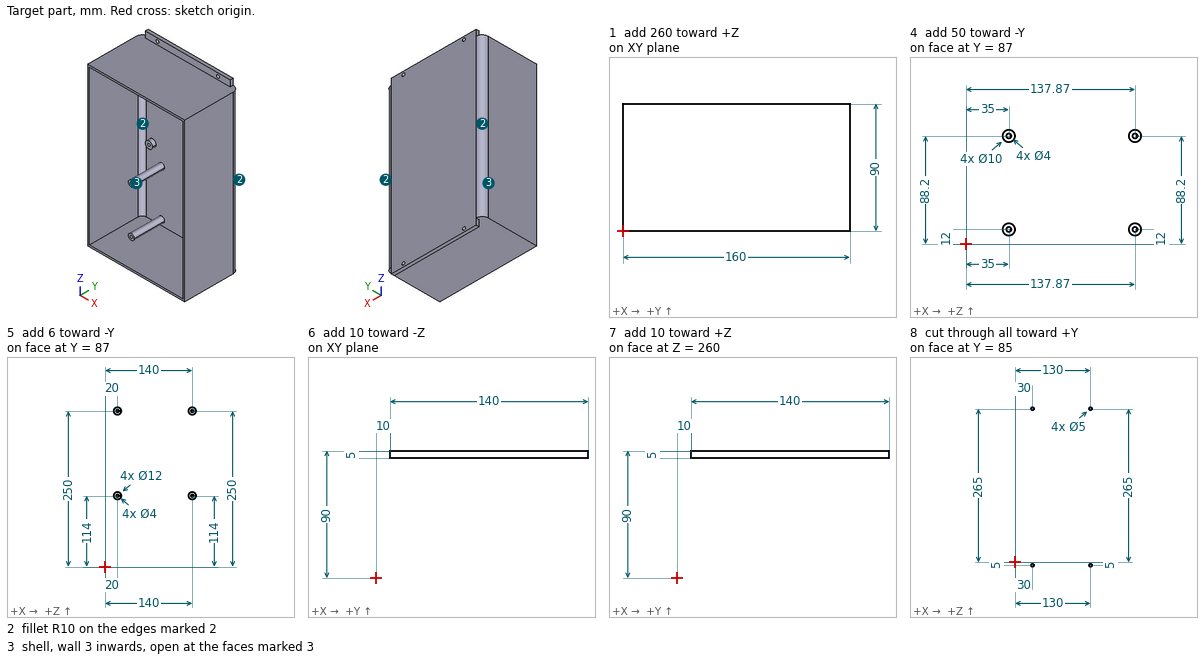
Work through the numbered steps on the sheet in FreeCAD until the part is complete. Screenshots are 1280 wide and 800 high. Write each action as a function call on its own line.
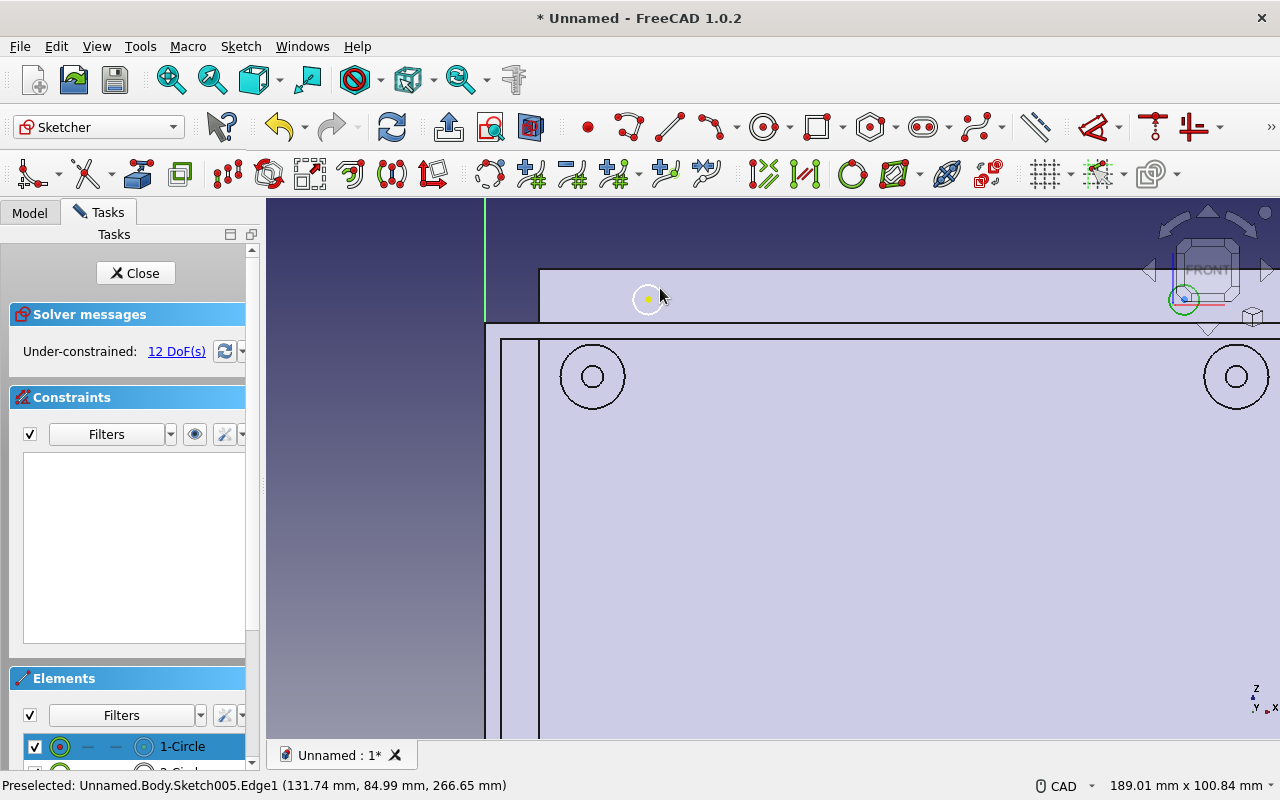
click(658, 289)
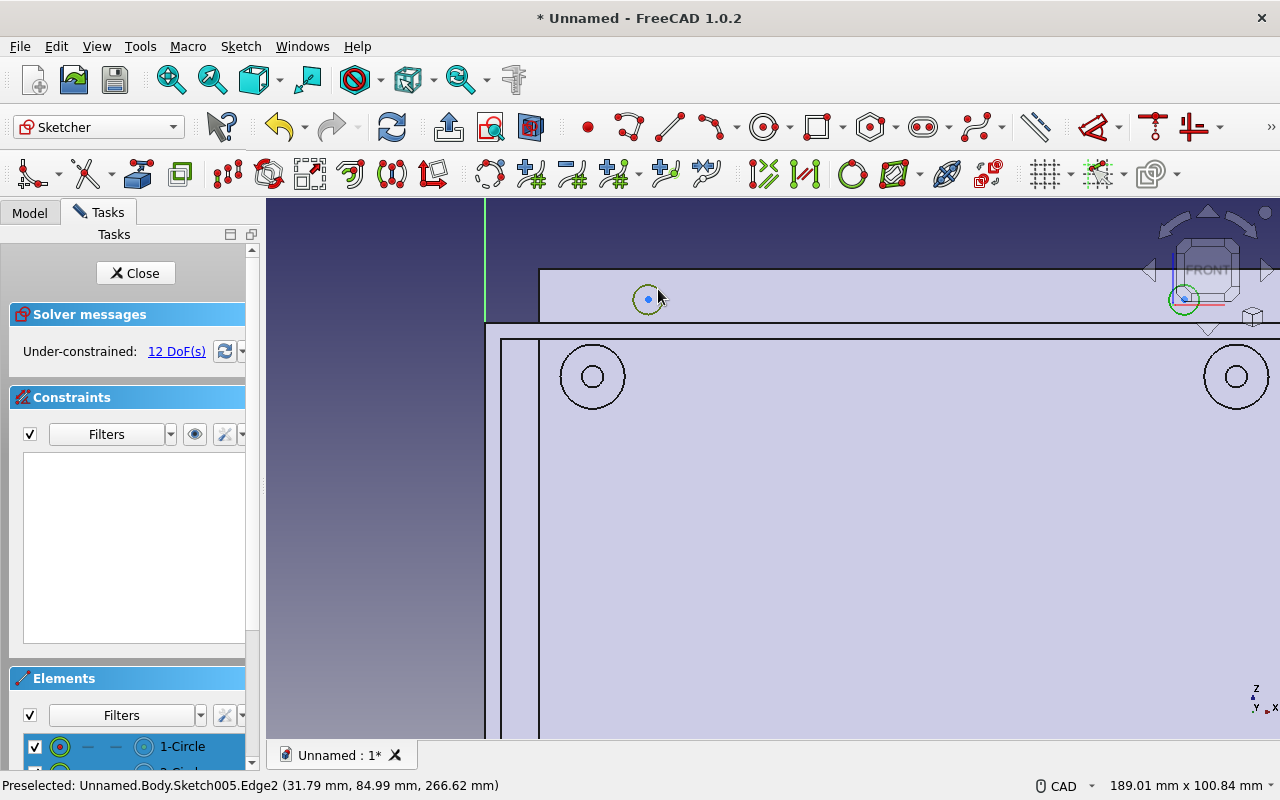
scroll(660, 288, down, 7)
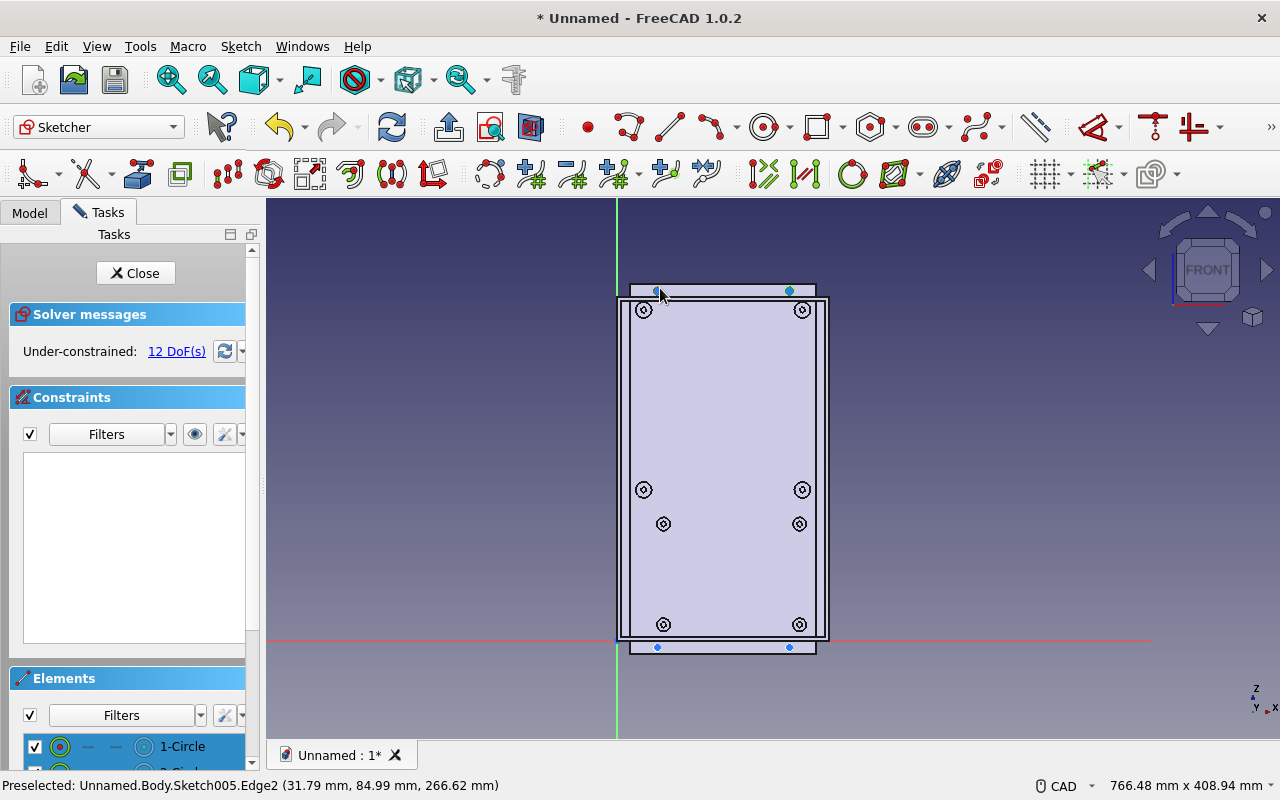
scroll(792, 645, up, 8)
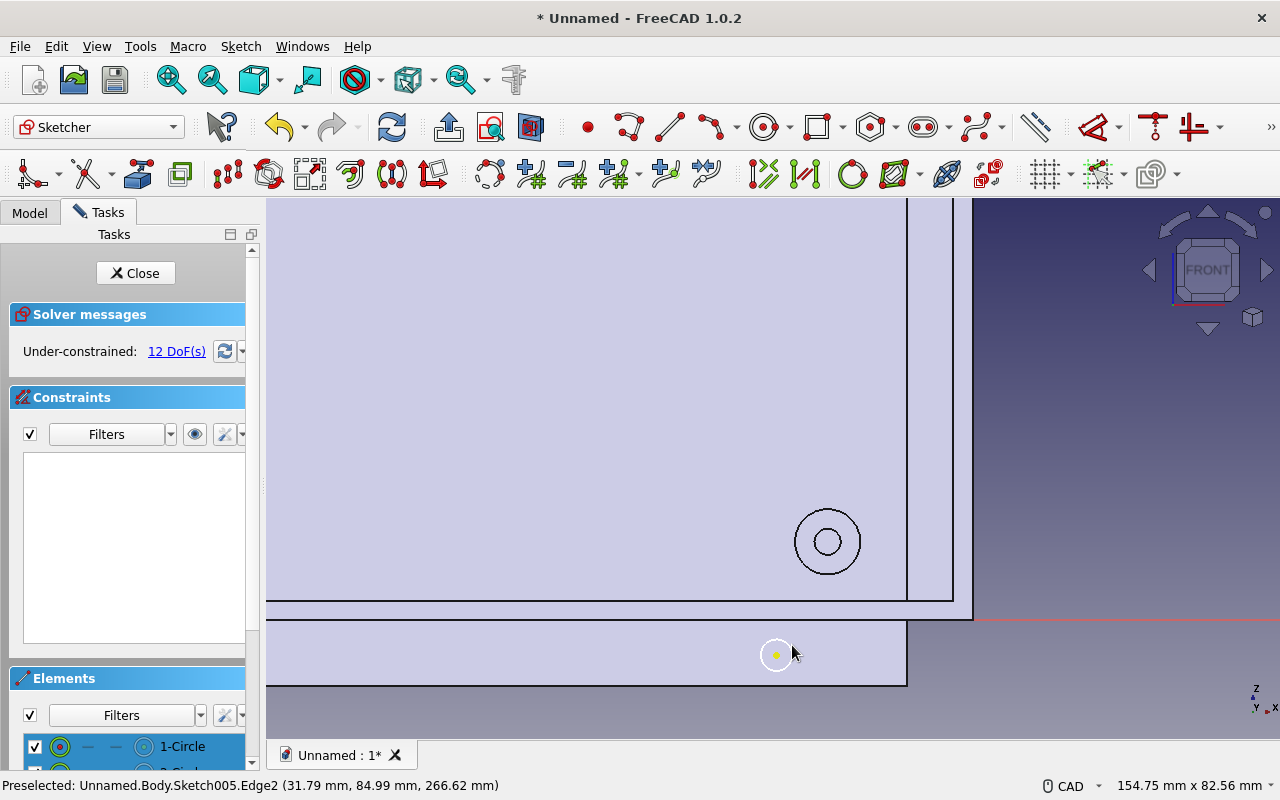
click(788, 644)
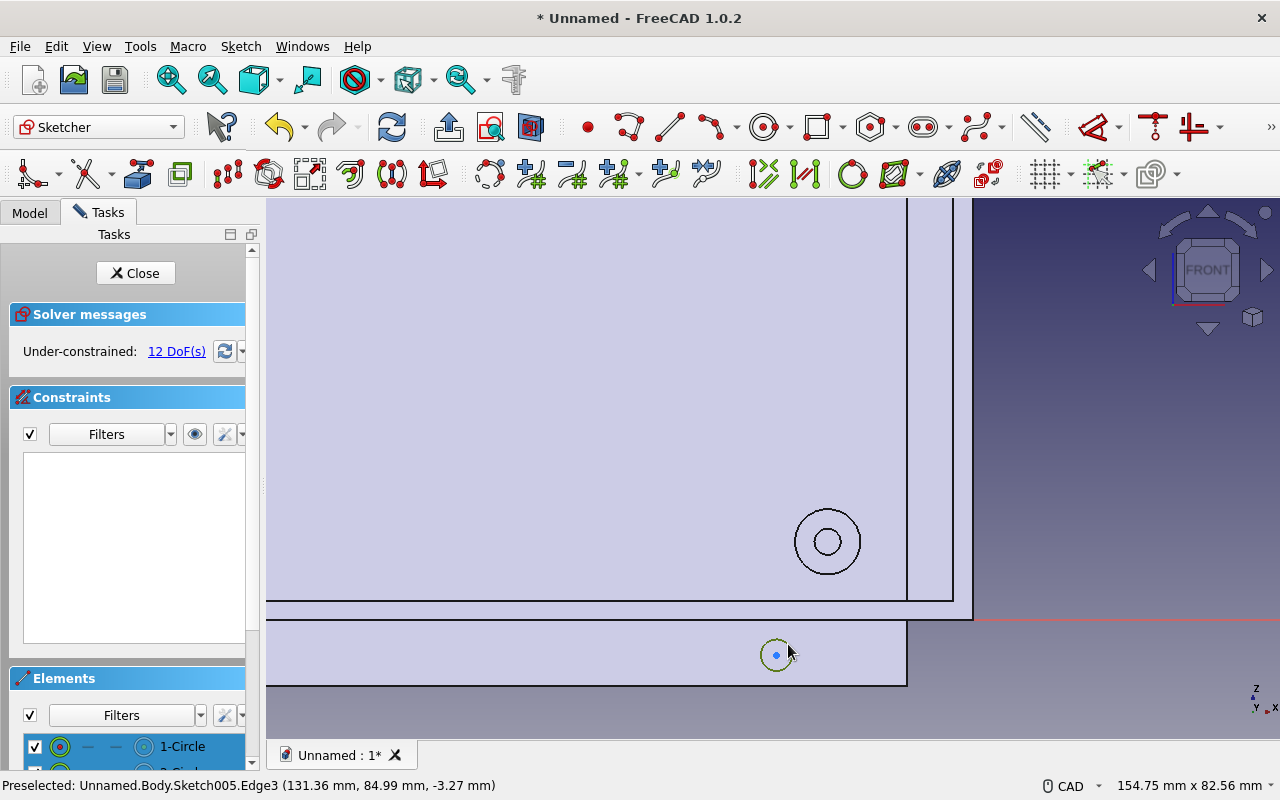
scroll(792, 646, down, 8)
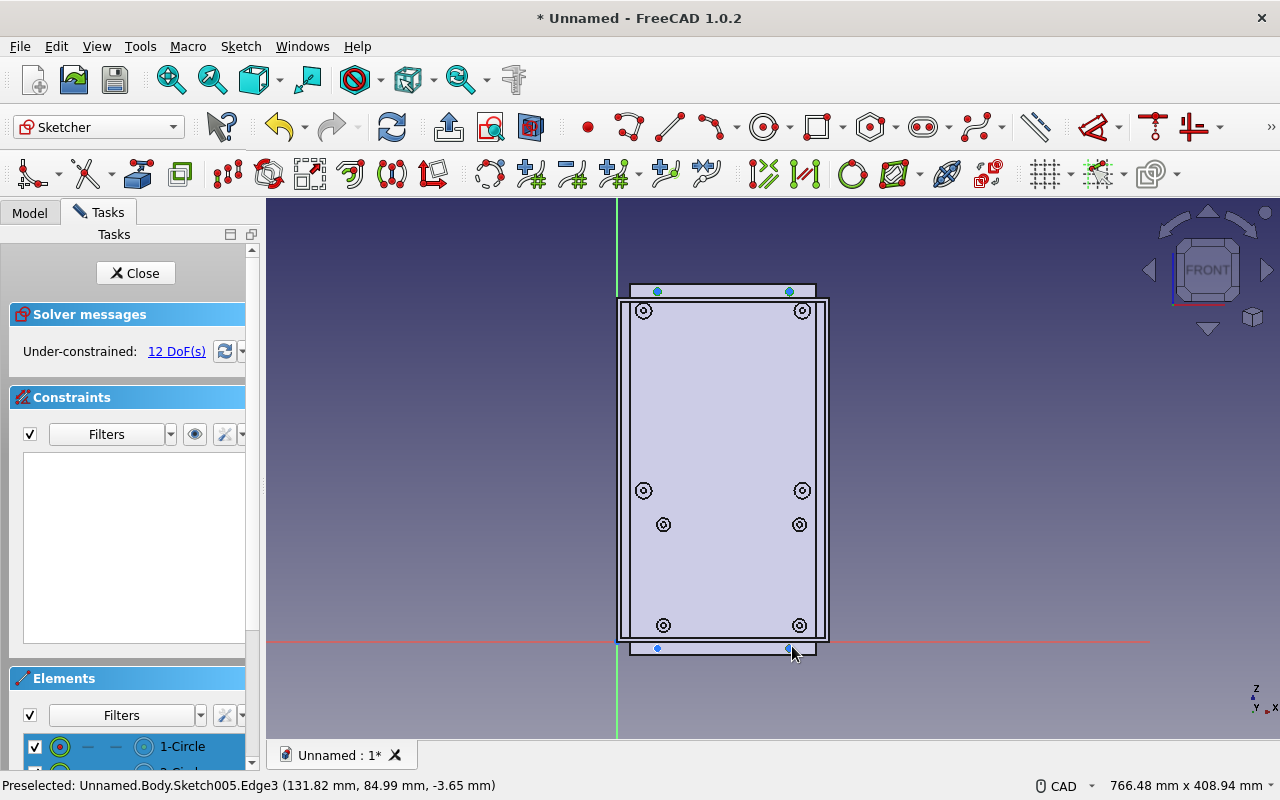
scroll(659, 646, up, 8)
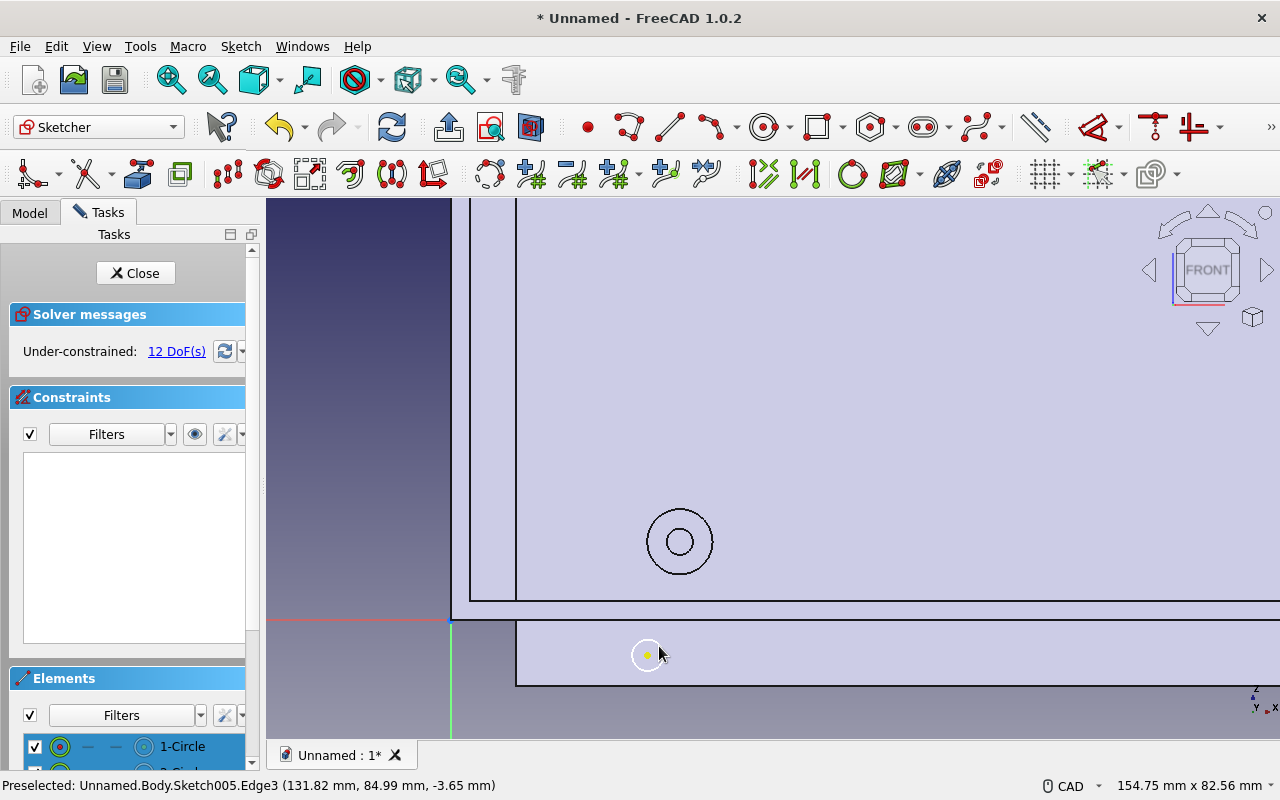
click(659, 644)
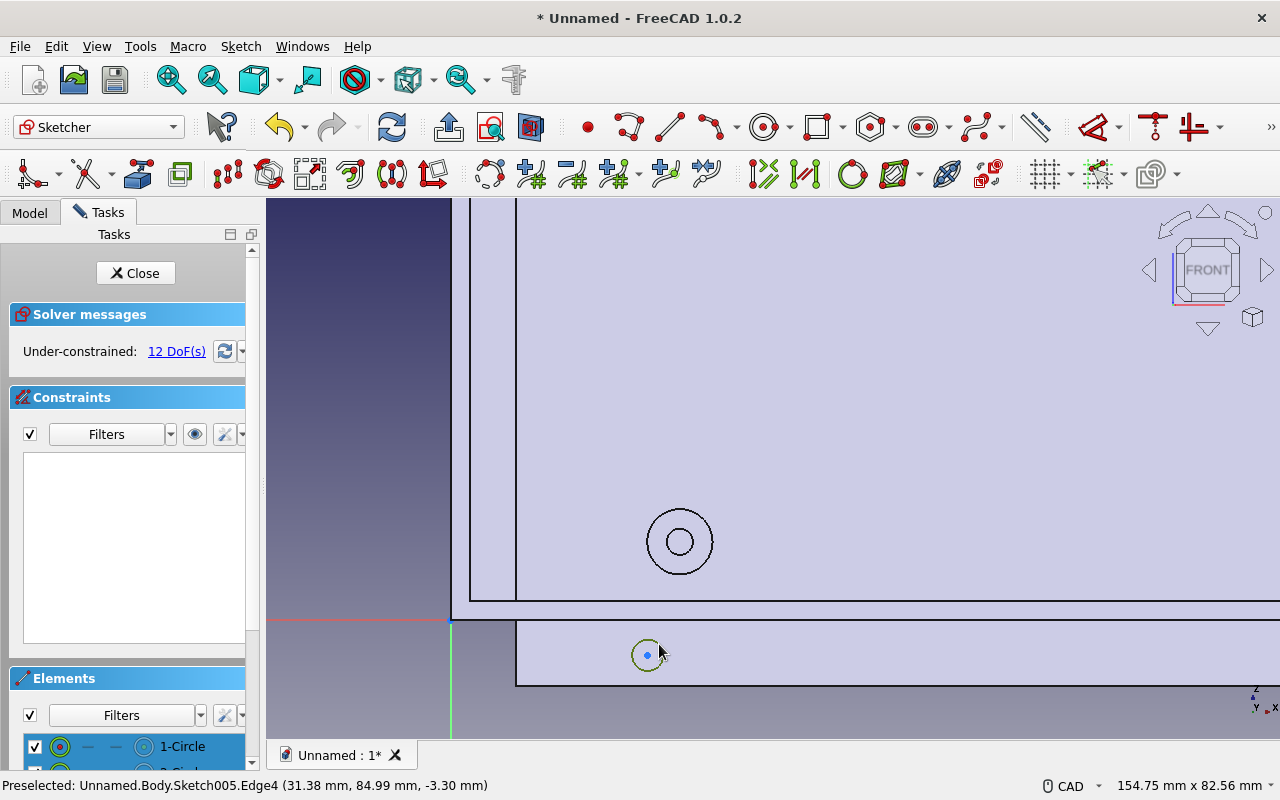
key(e)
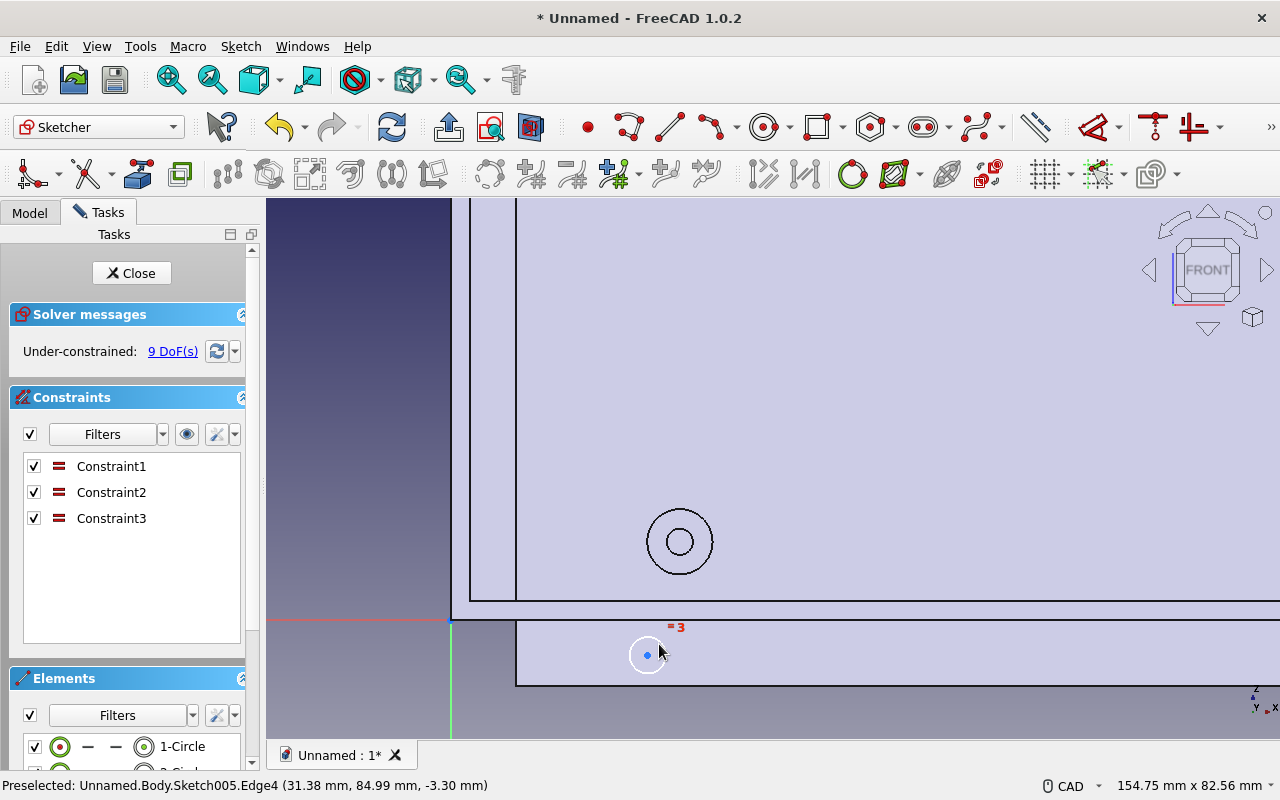
click(1092, 128)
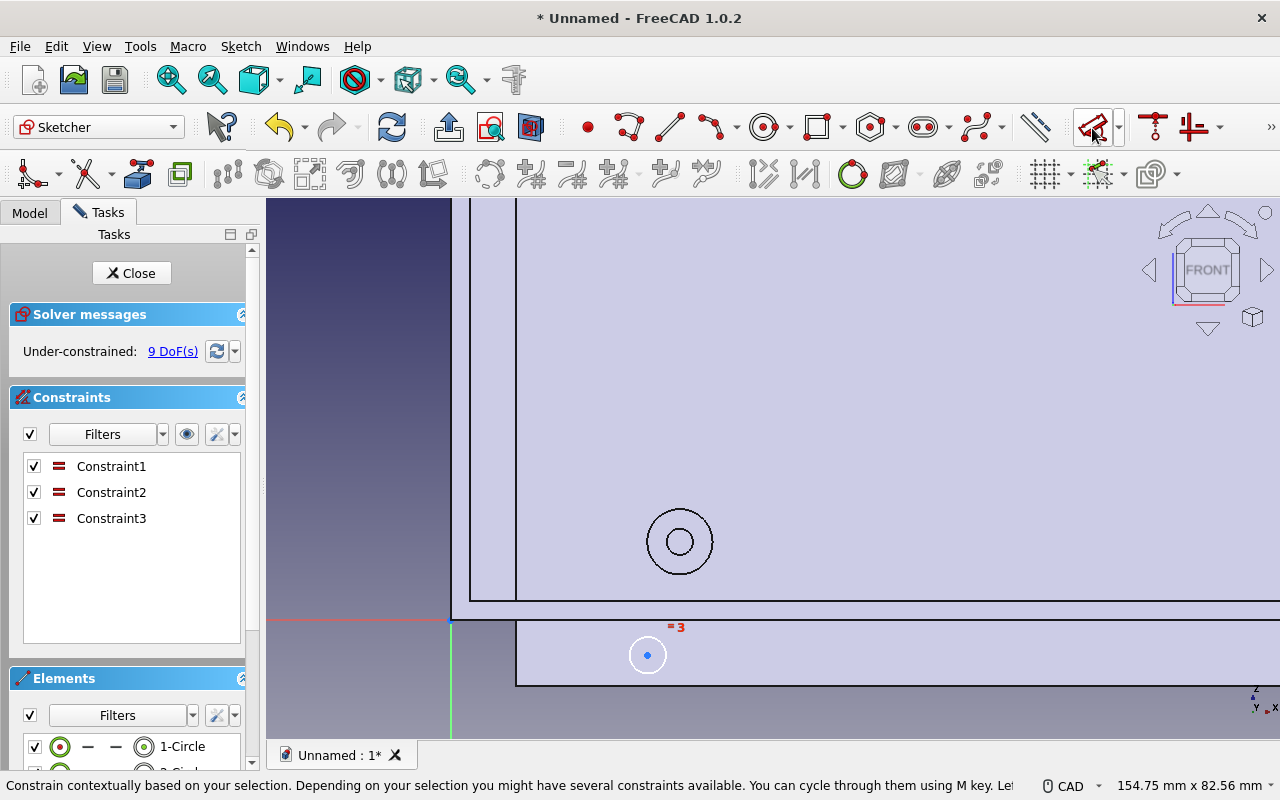
scroll(659, 646, down, 8)